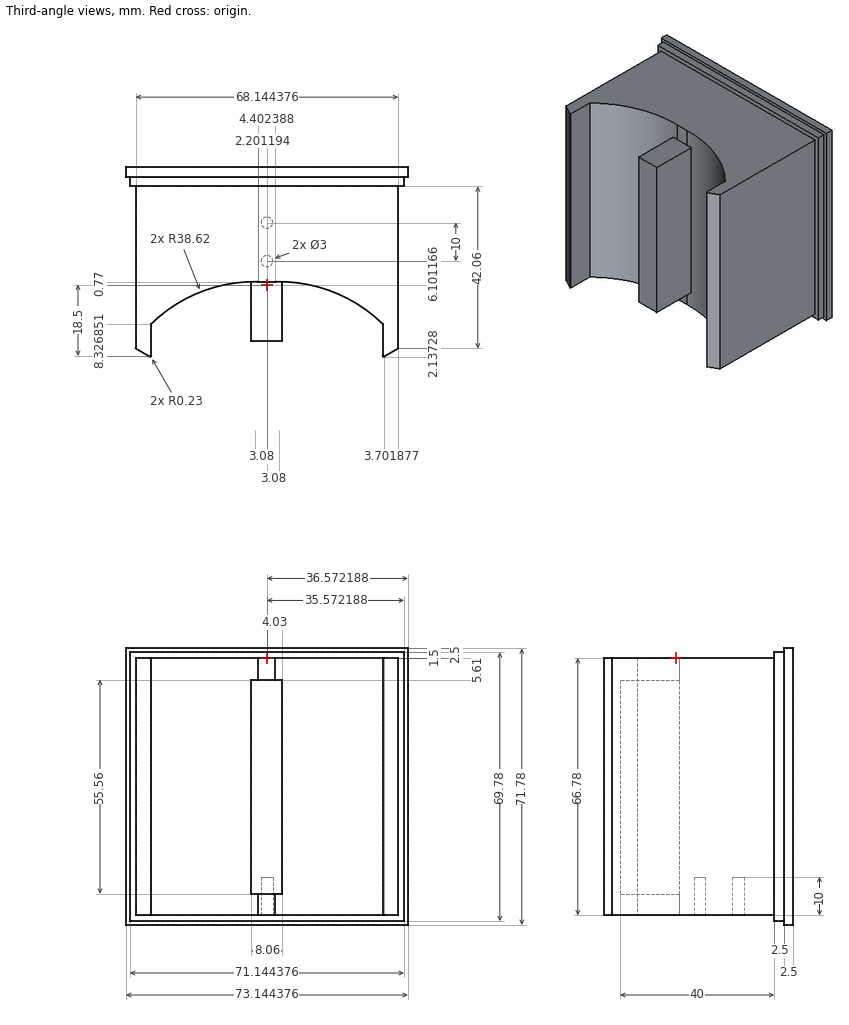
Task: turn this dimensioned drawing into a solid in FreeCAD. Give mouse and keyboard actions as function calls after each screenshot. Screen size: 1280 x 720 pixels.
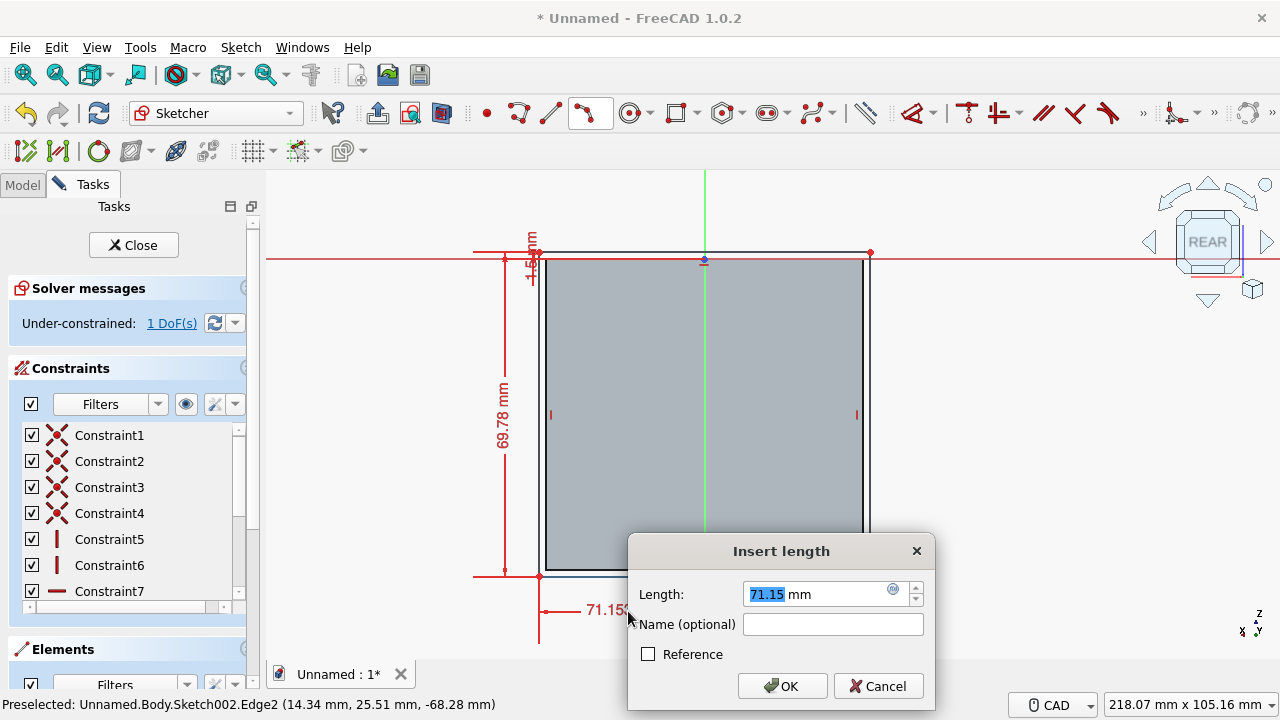
text(71.144376)
key(Return)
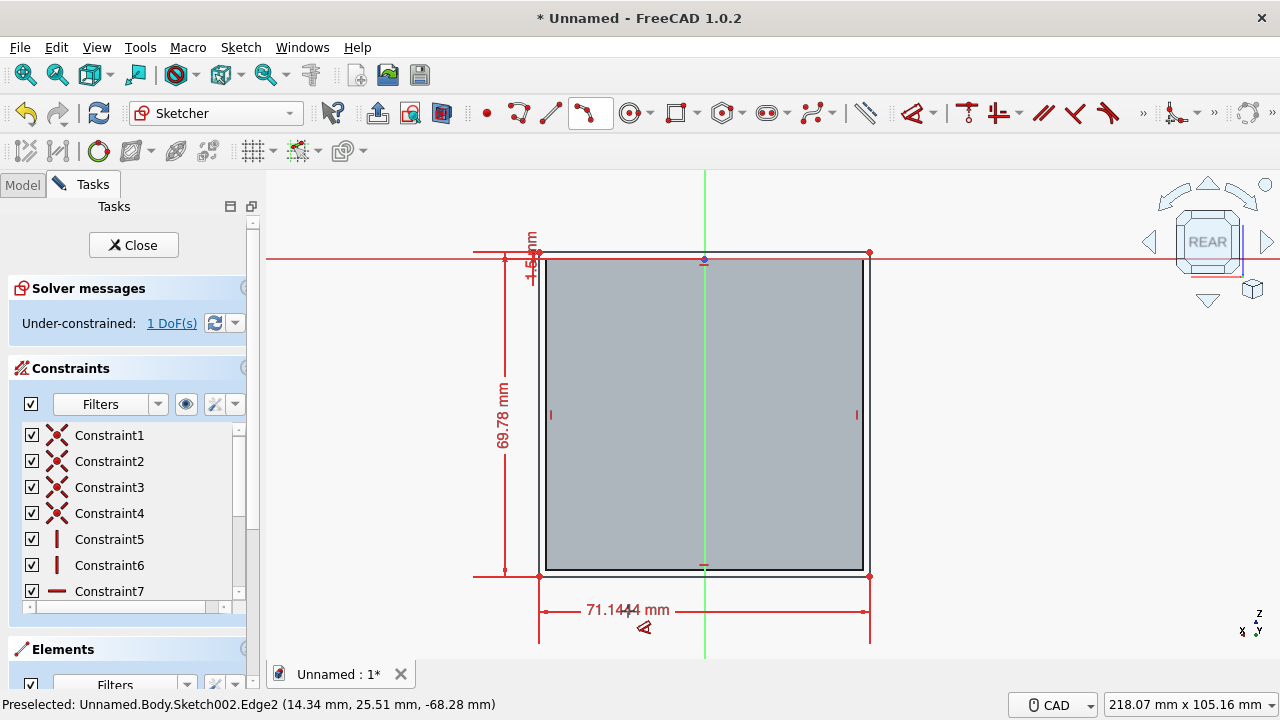
click(539, 252)
click(622, 218)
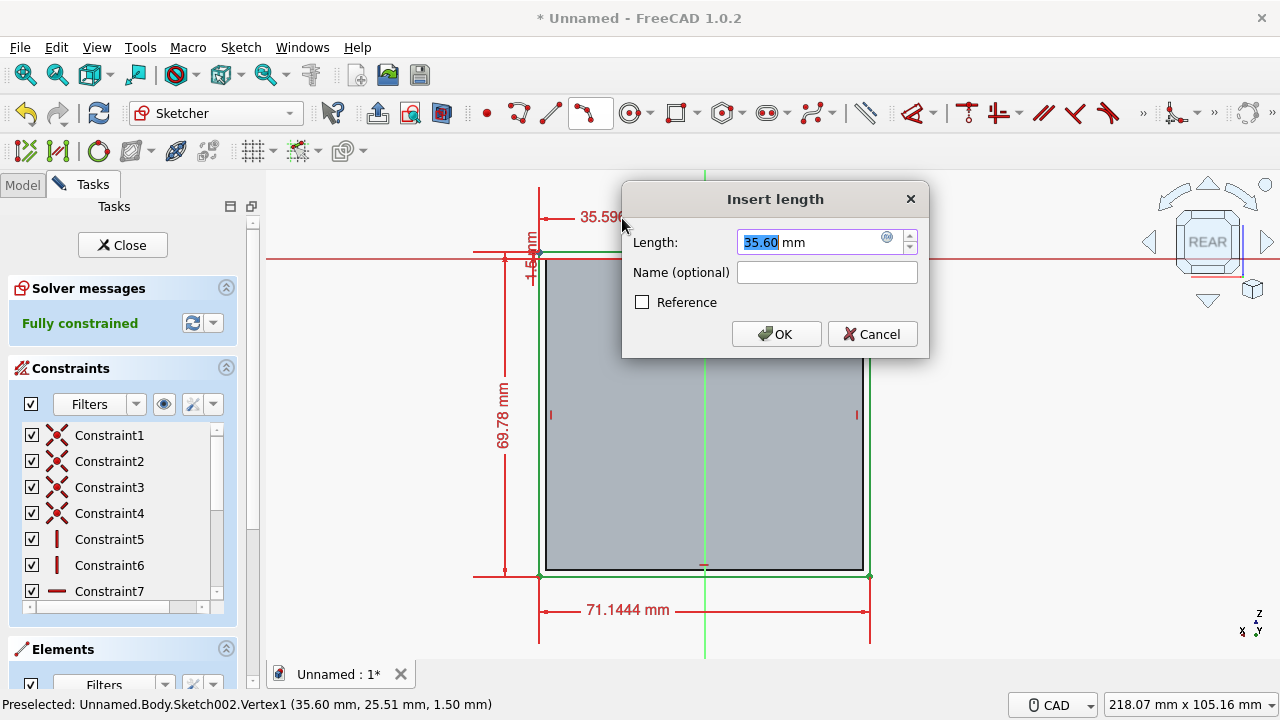
text(35.572188)
key(Return)
key(Escape)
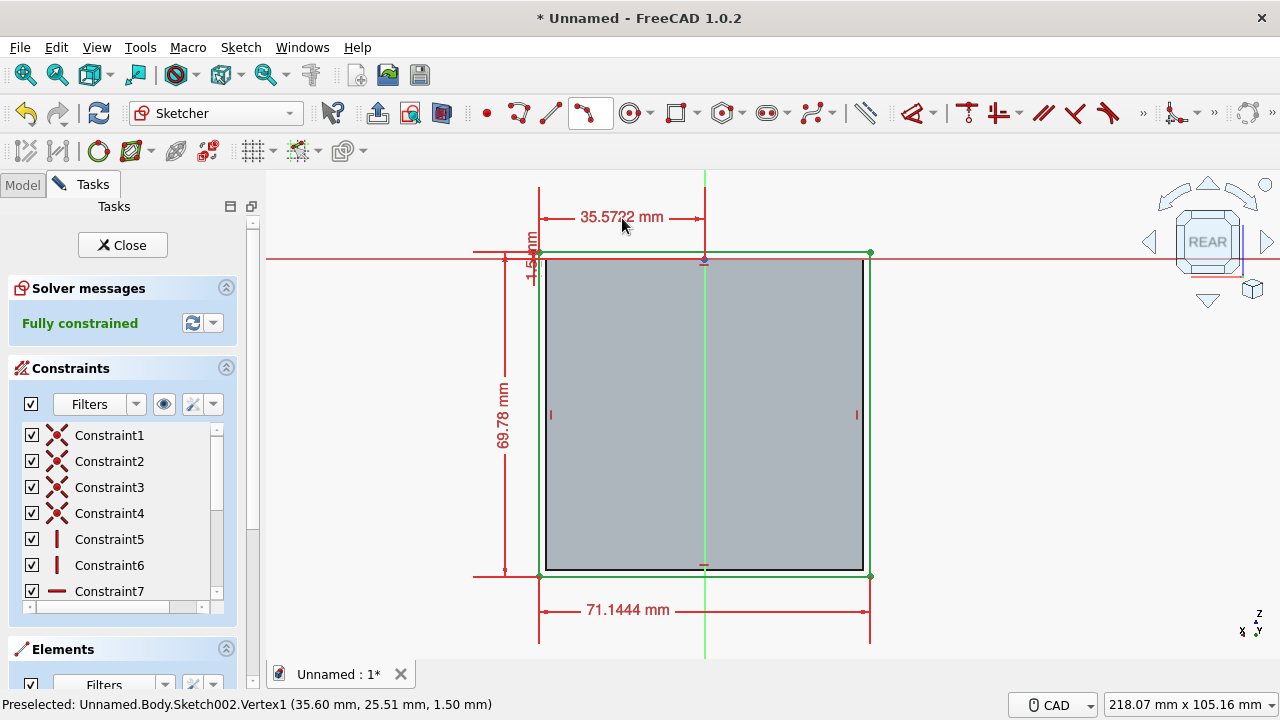
click(123, 245)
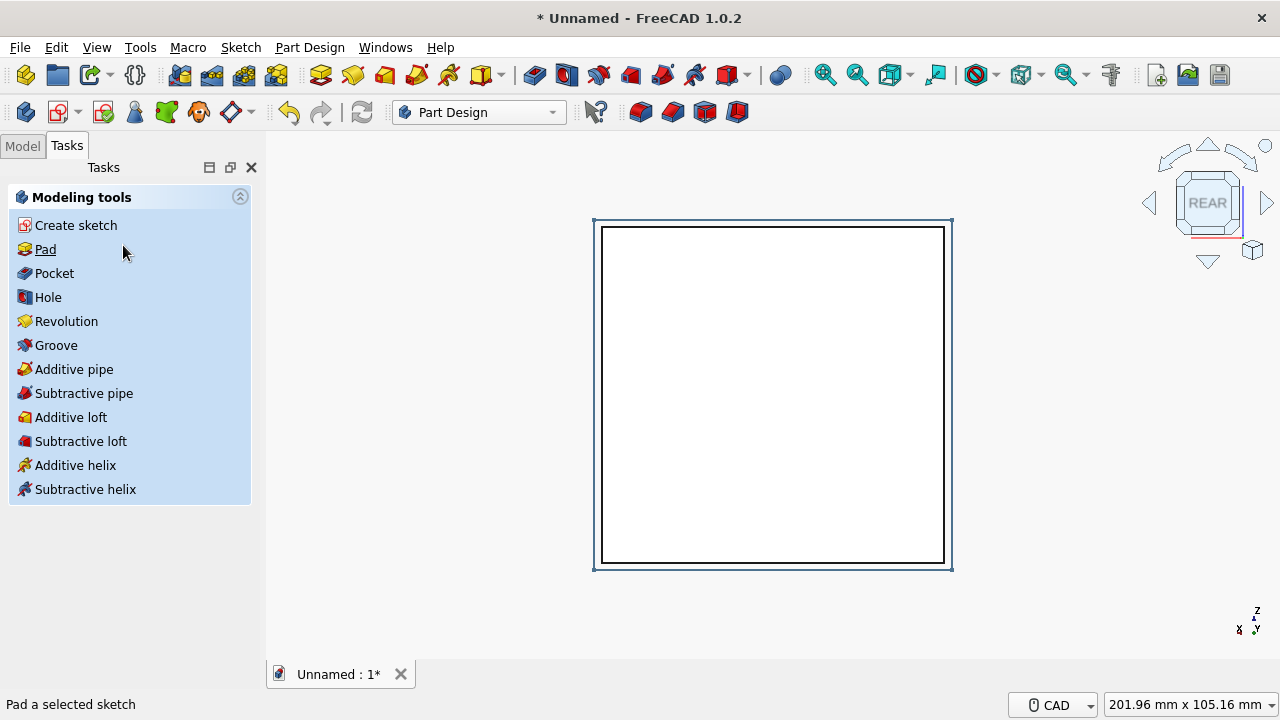
click(322, 76)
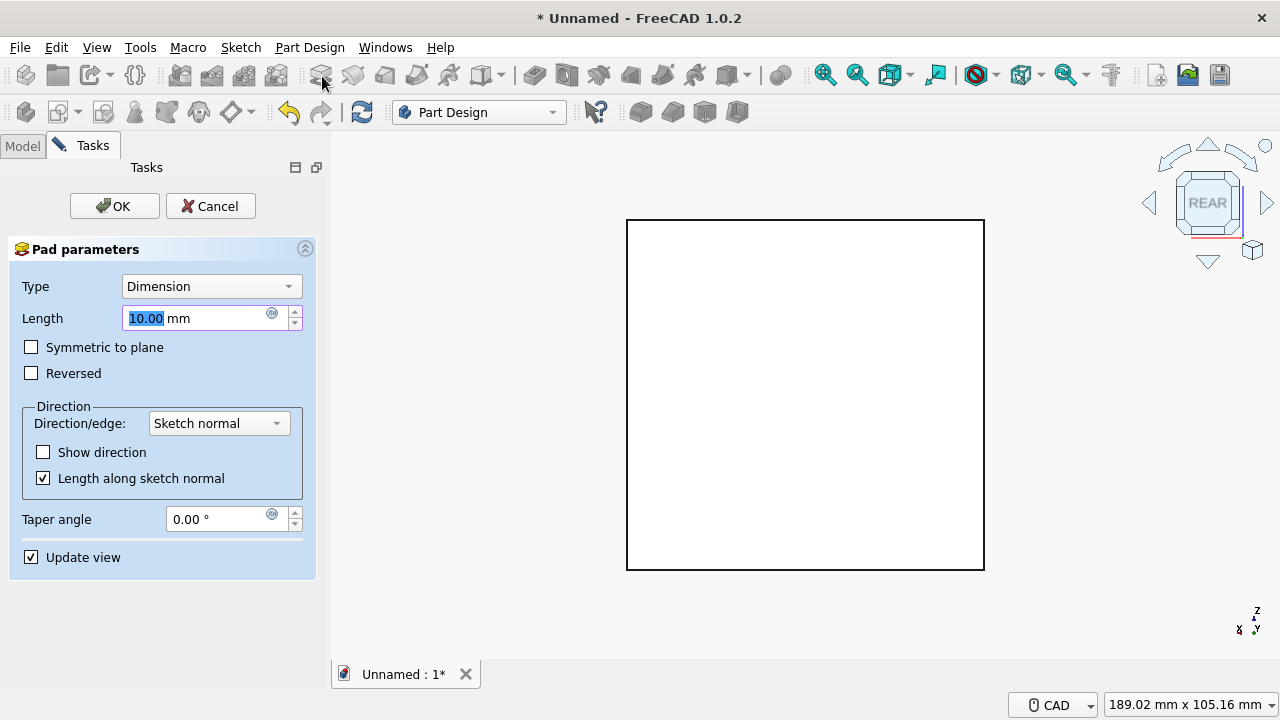
text(2.5)
key(Tab)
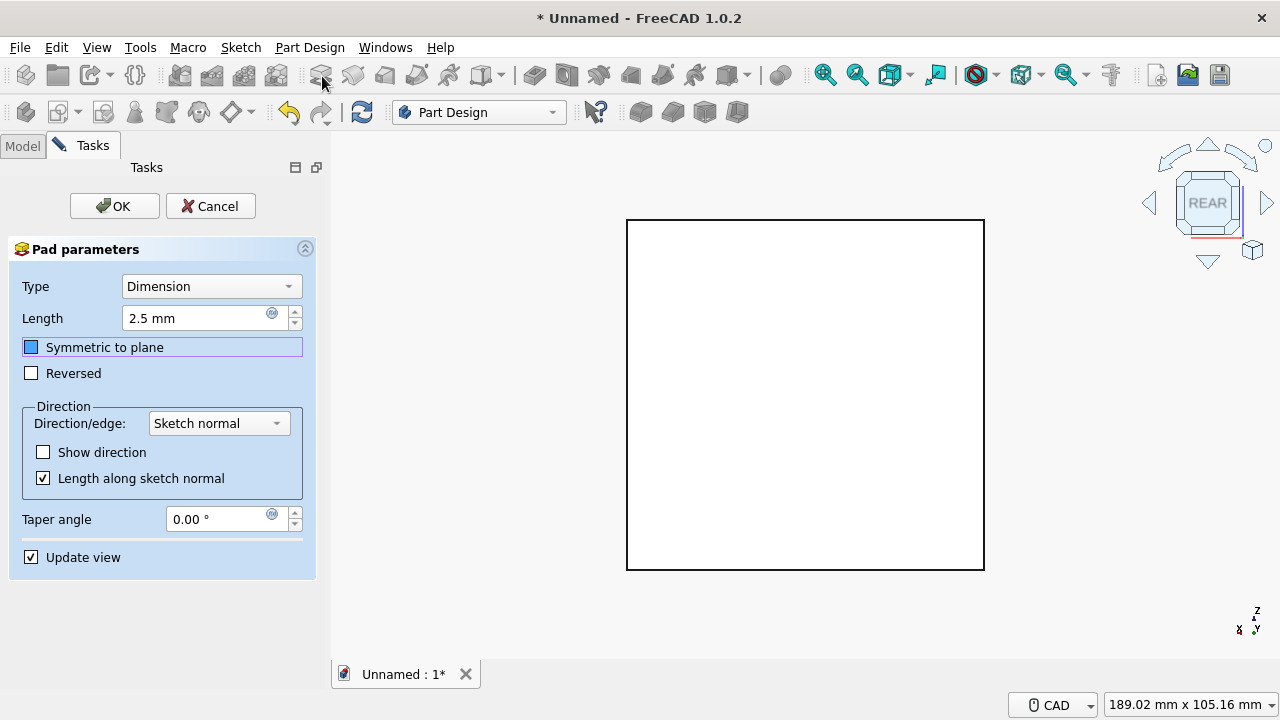
click(115, 206)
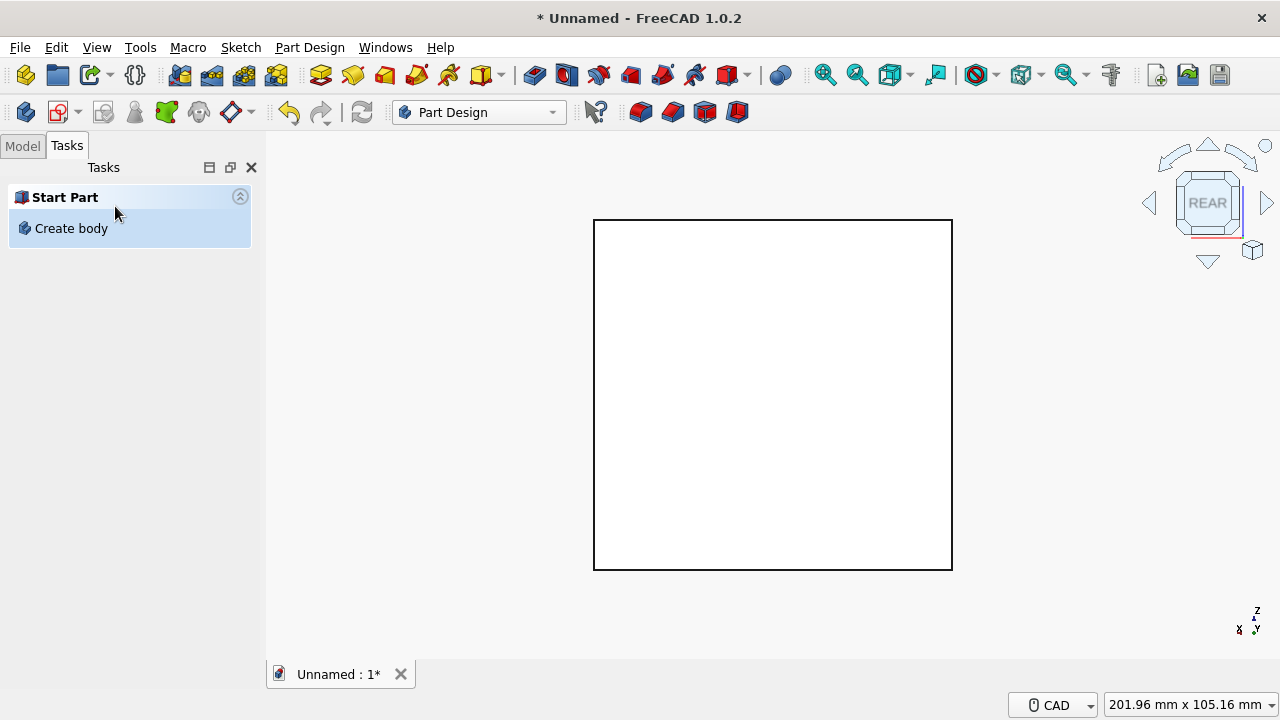
click(773, 394)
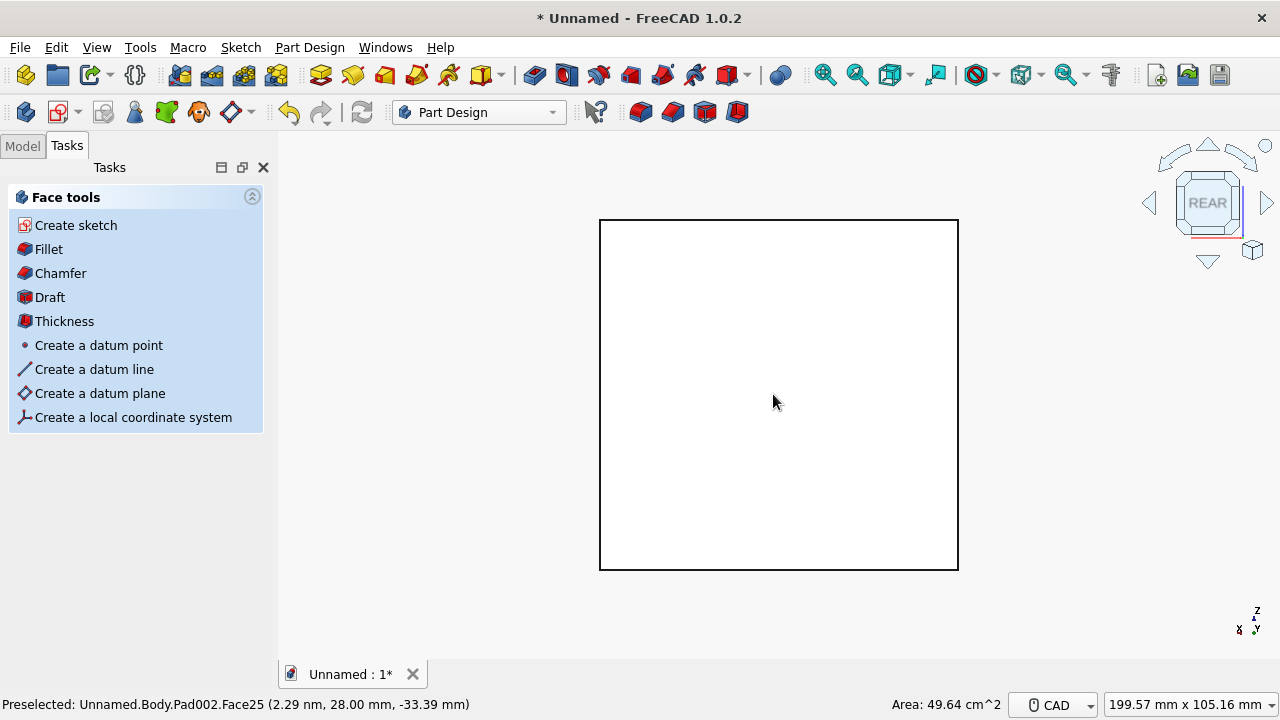
click(58, 112)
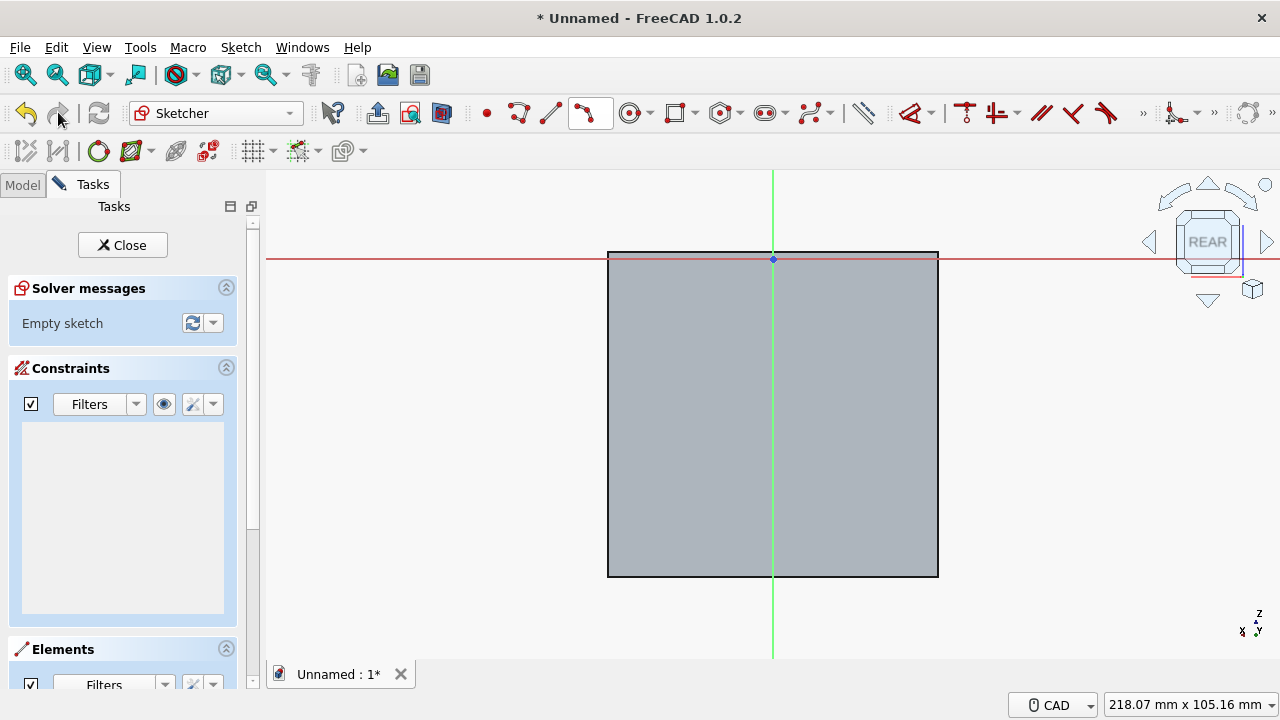
click(676, 114)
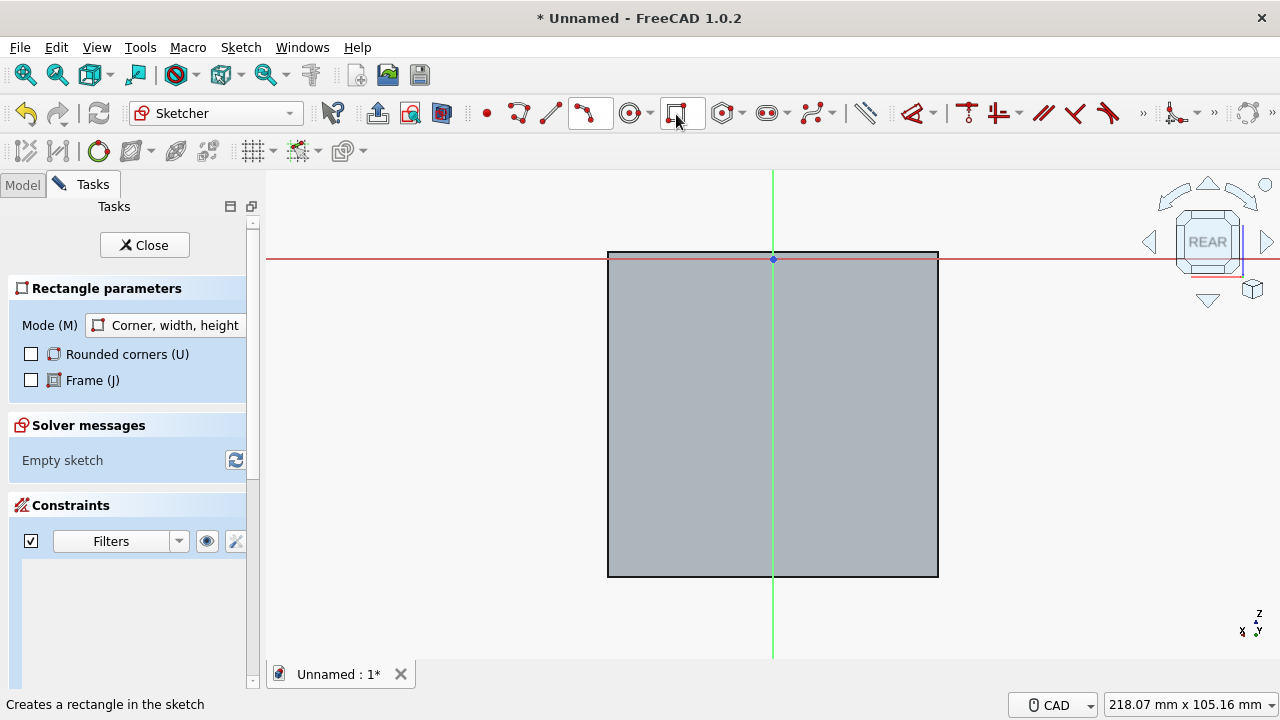
scroll(603, 248, up, 2)